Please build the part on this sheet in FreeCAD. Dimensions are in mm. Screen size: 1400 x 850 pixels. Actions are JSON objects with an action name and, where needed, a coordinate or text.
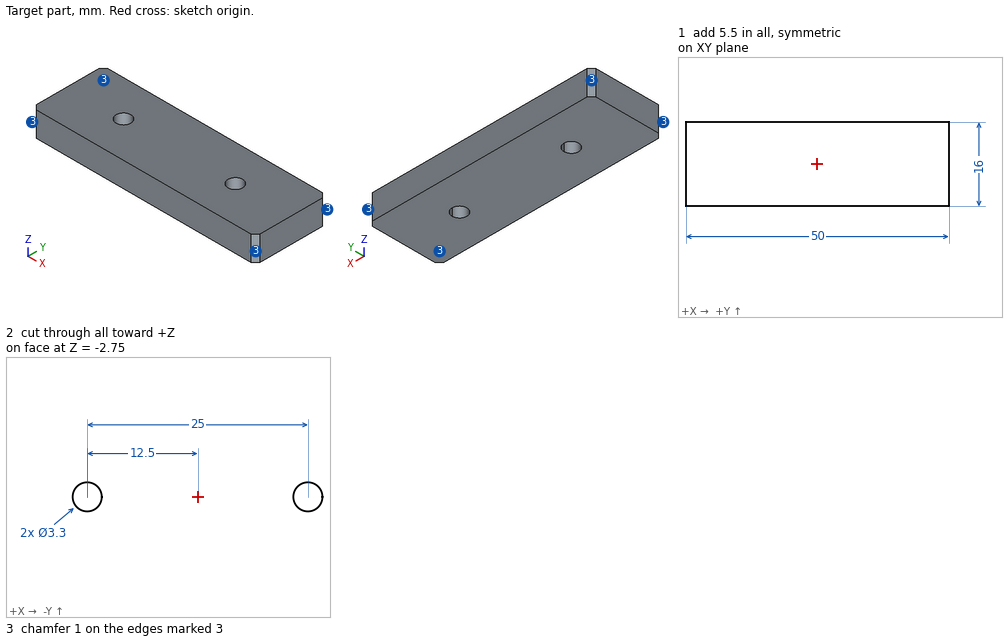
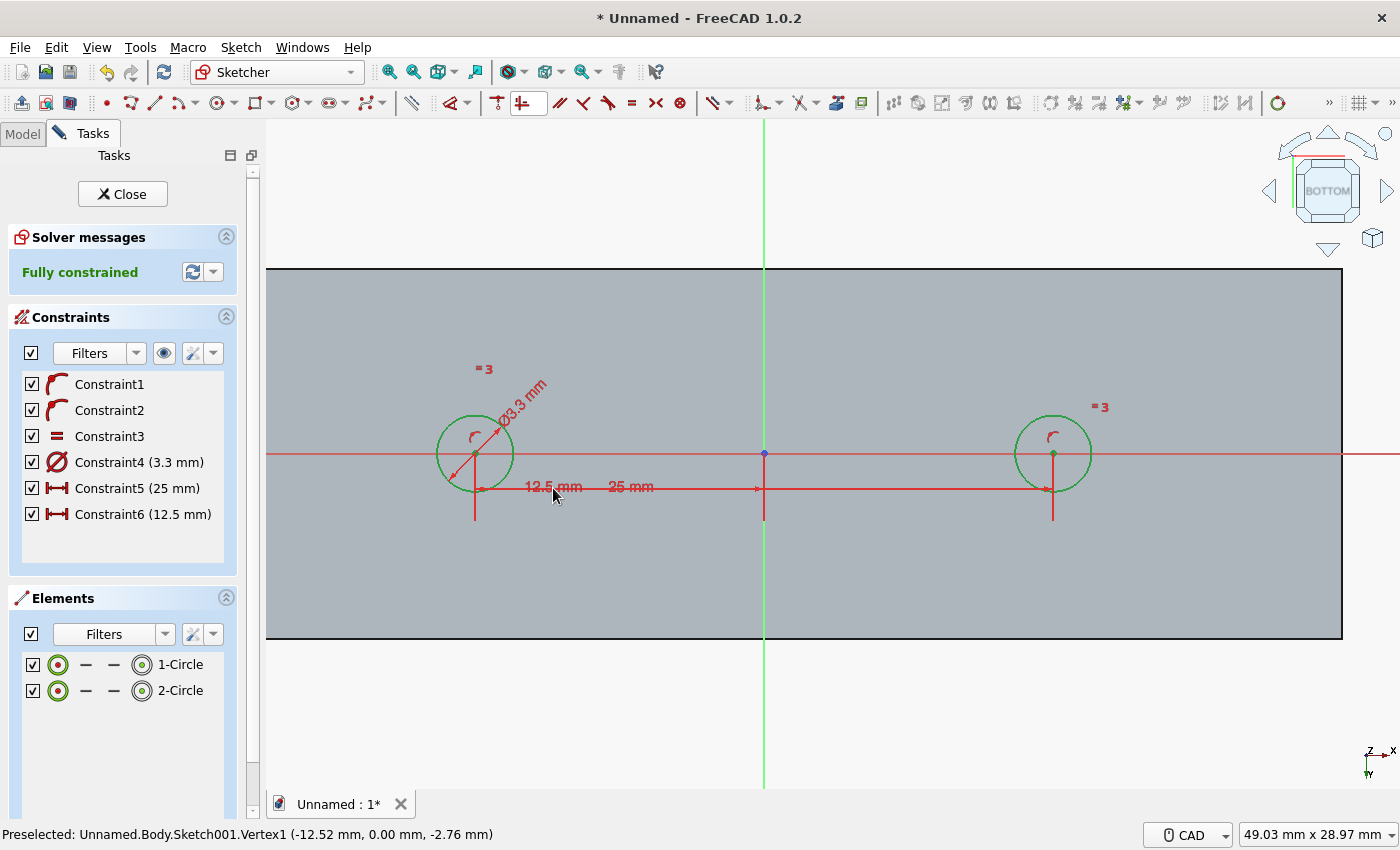
{"action": "left_click", "coordinate": [123, 194]}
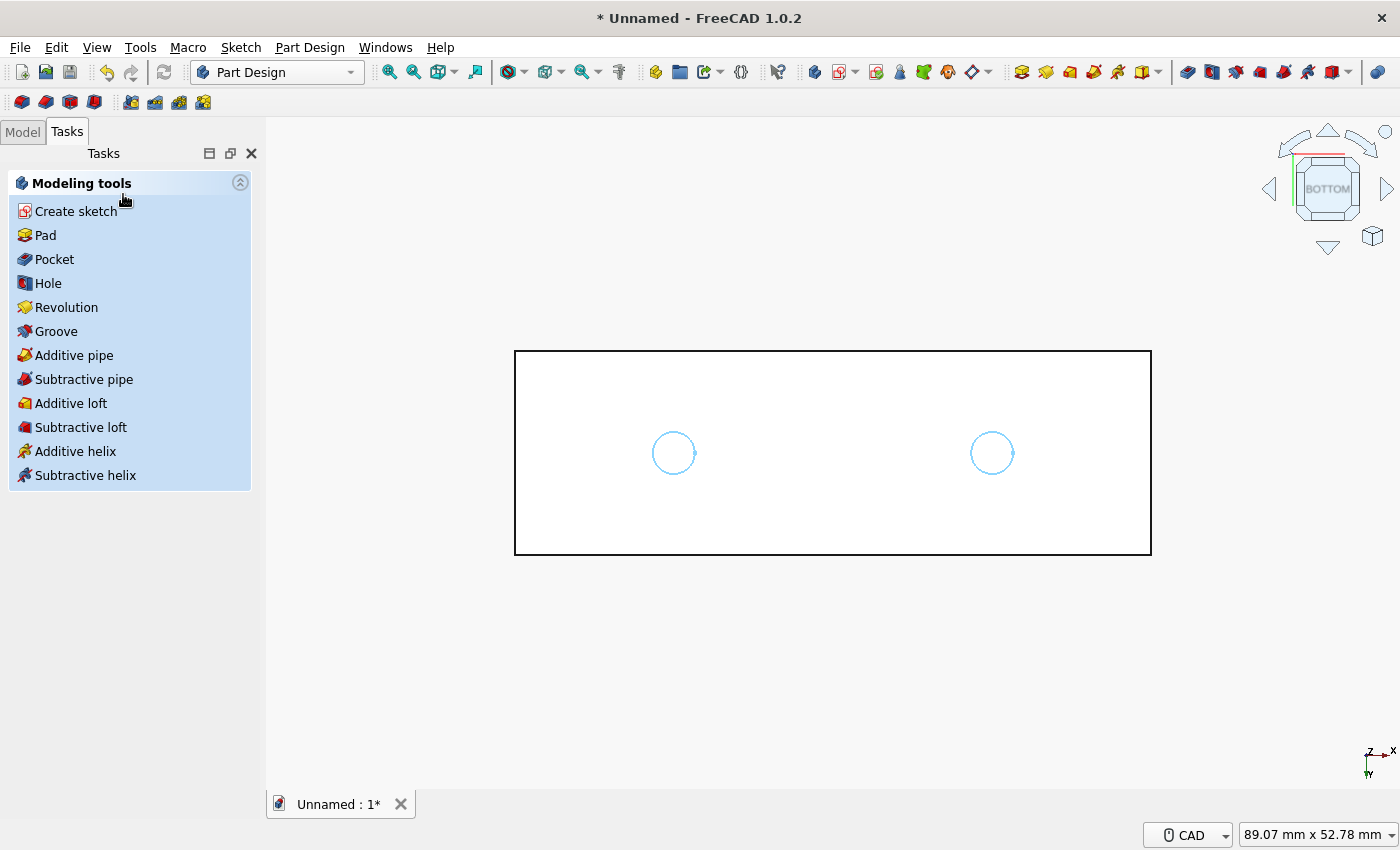
{"action": "left_click", "coordinate": [1188, 72]}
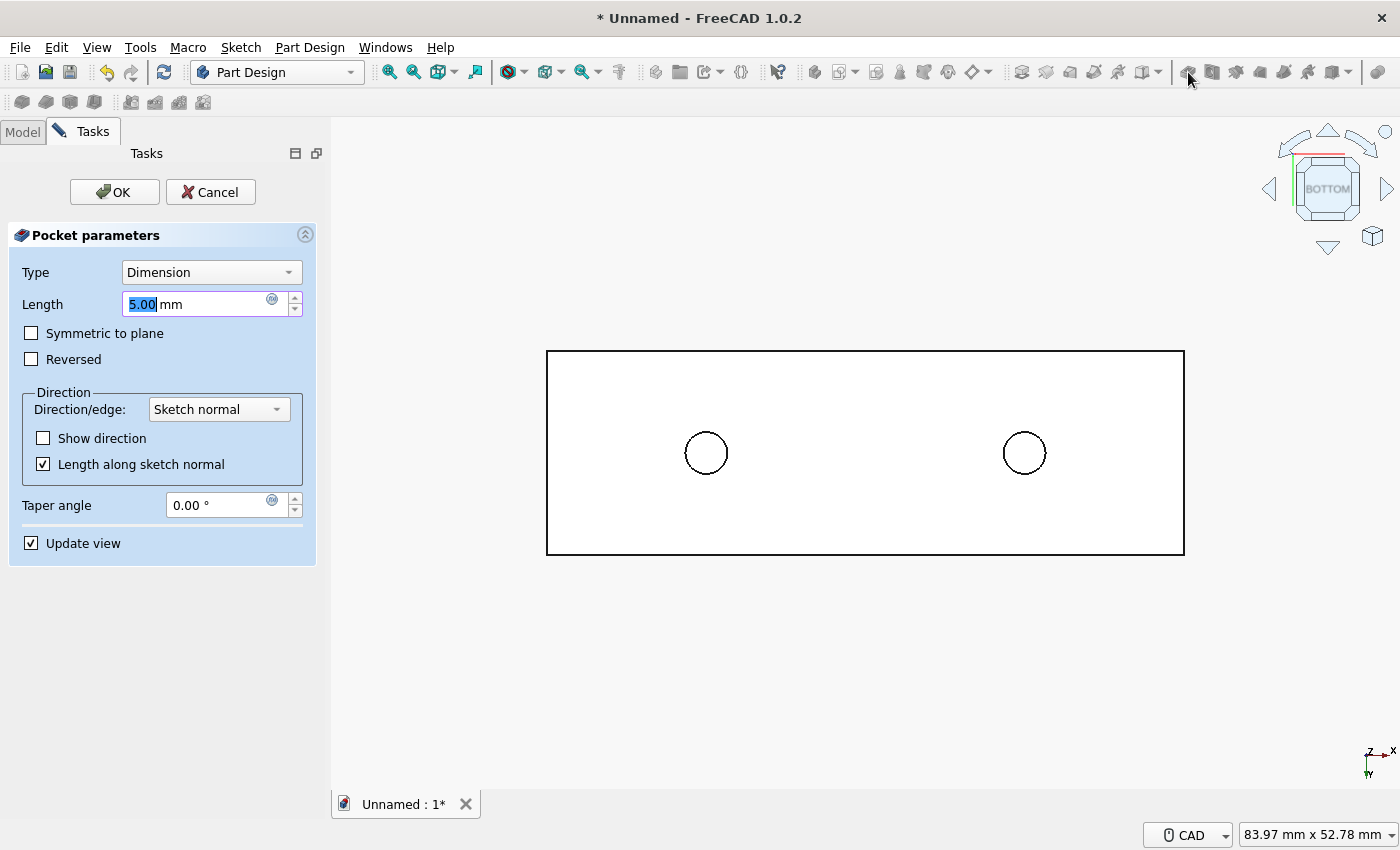
{"action": "left_click", "coordinate": [212, 272]}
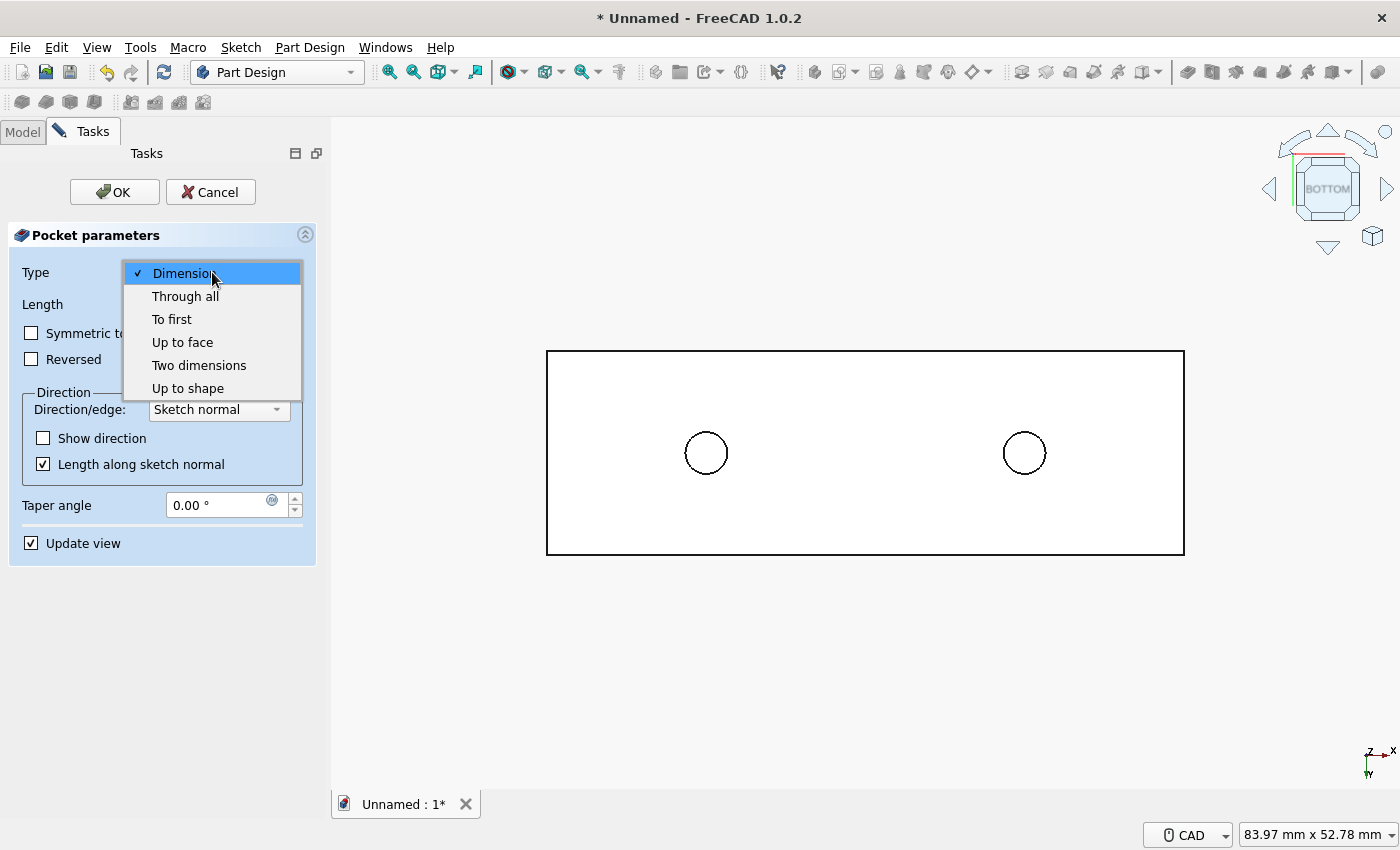
{"action": "left_click", "coordinate": [212, 296]}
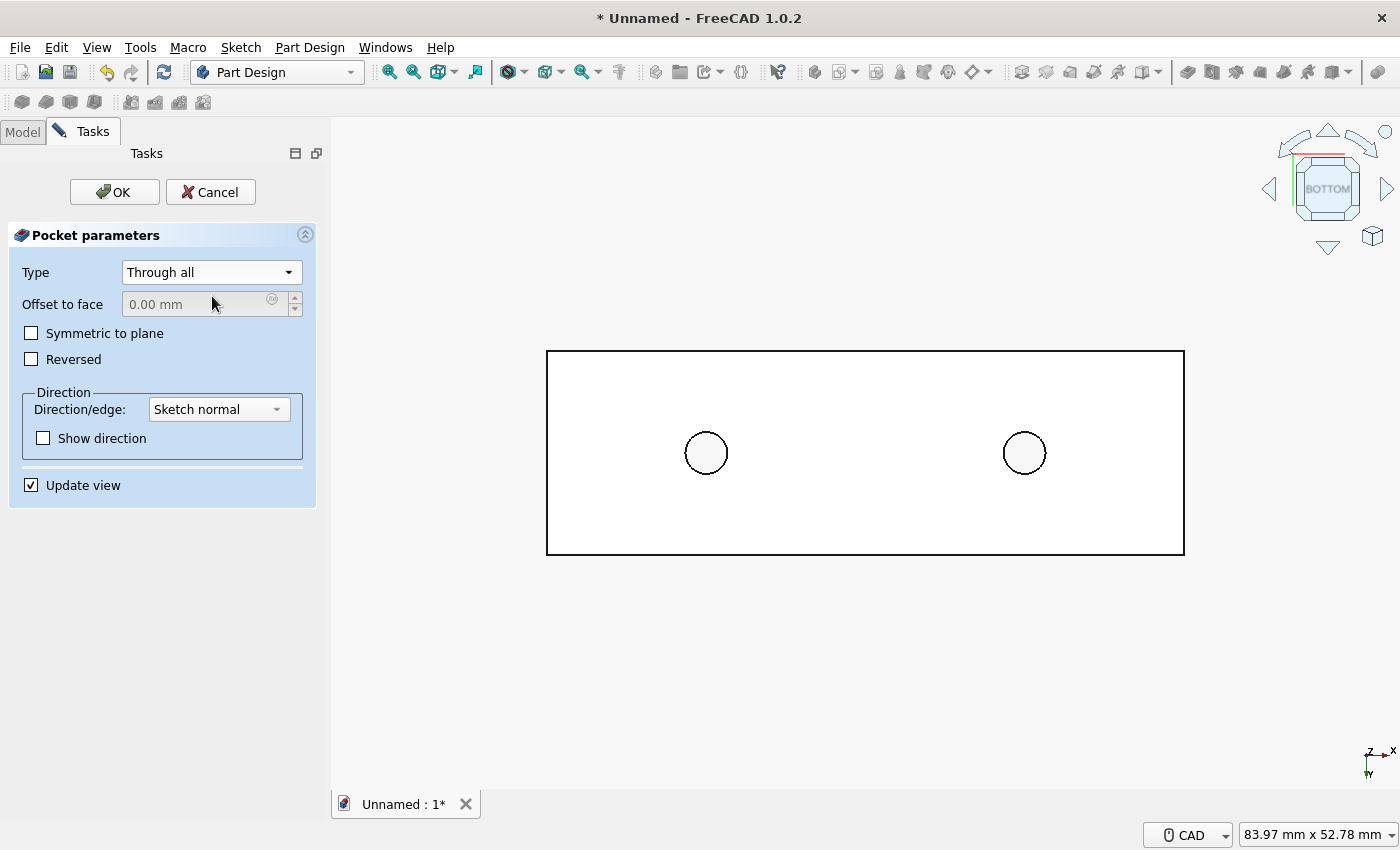
{"action": "left_click", "coordinate": [115, 192]}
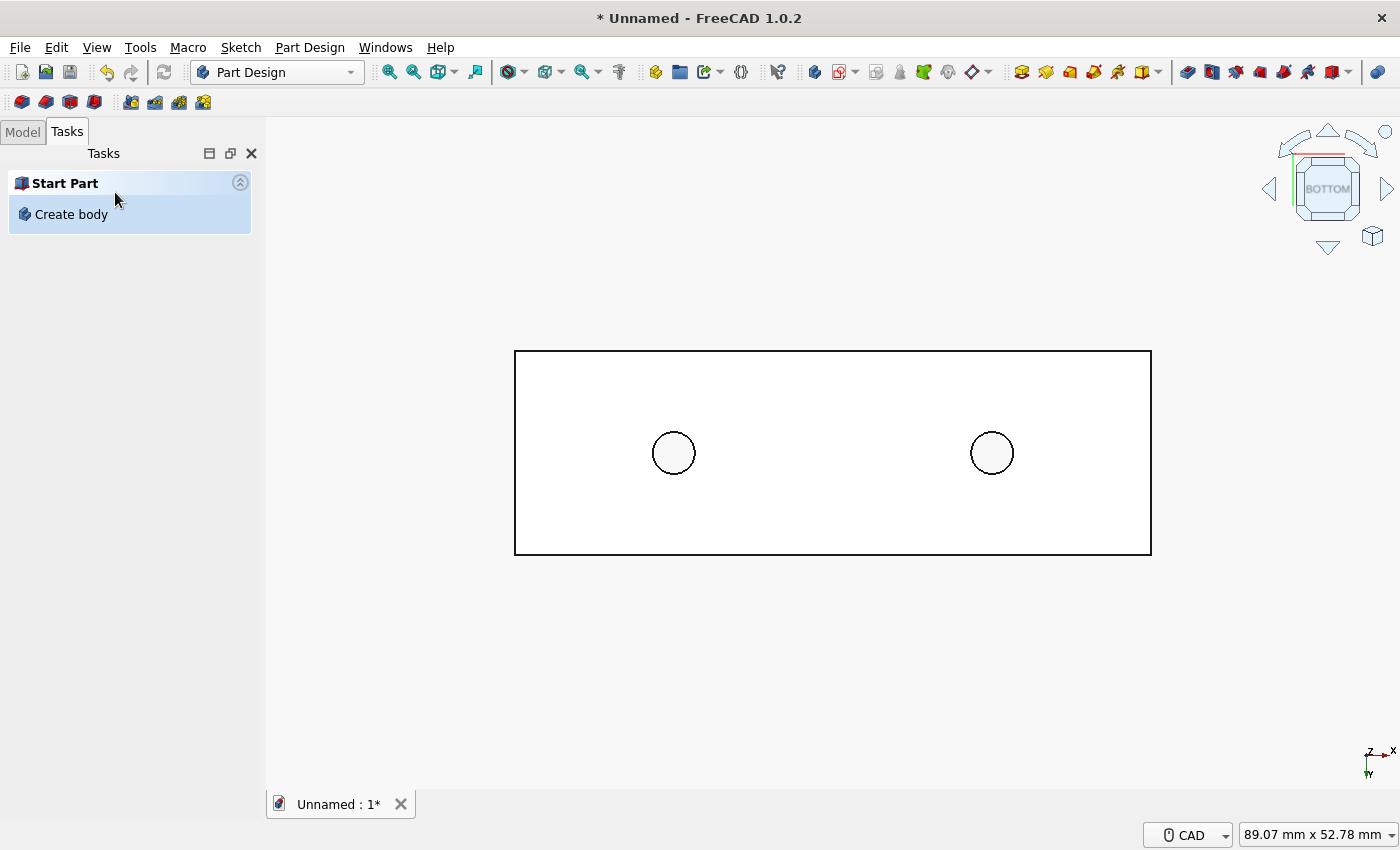
{"action": "key", "text": "0"}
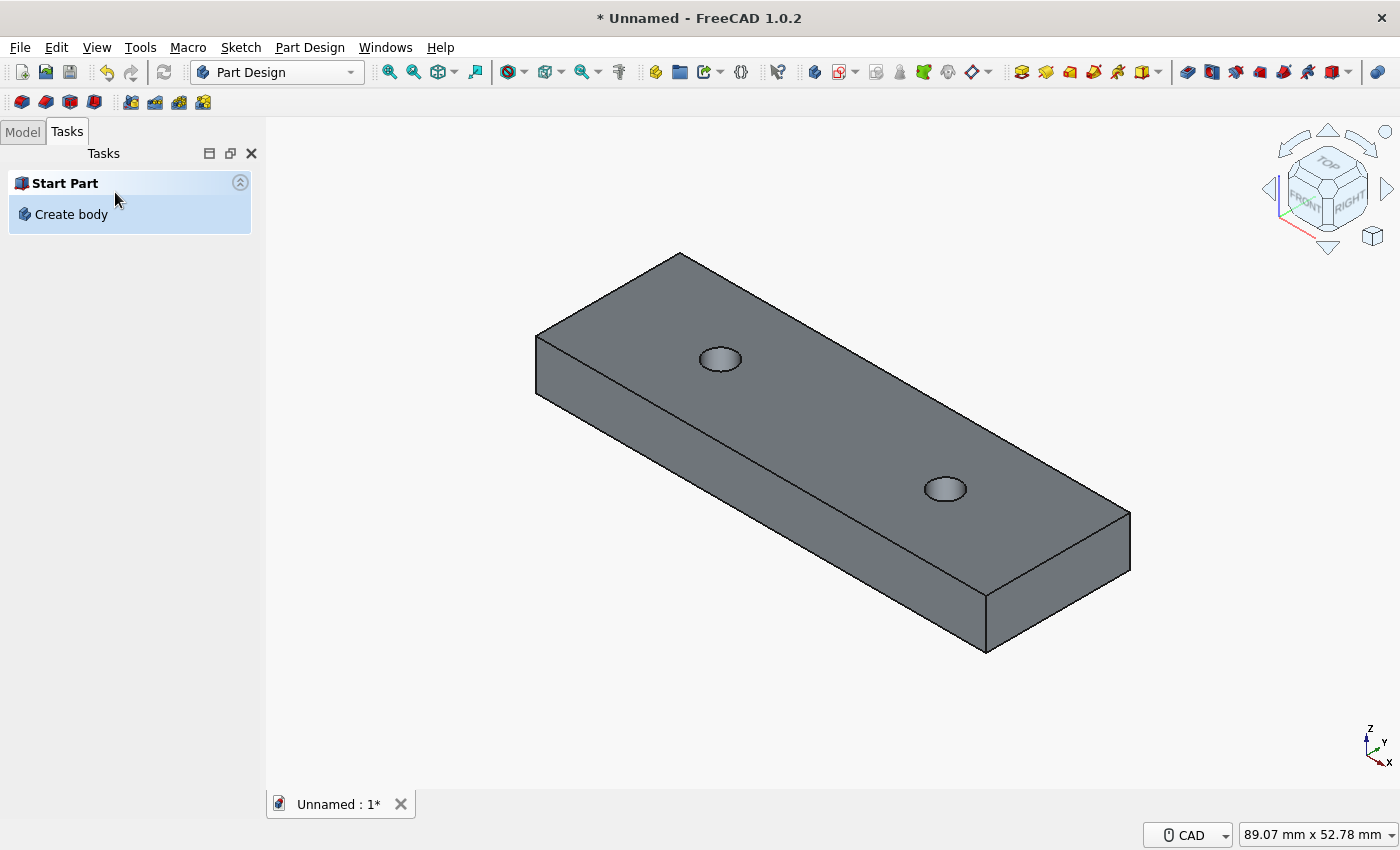
{"action": "left_click", "coordinate": [986, 624]}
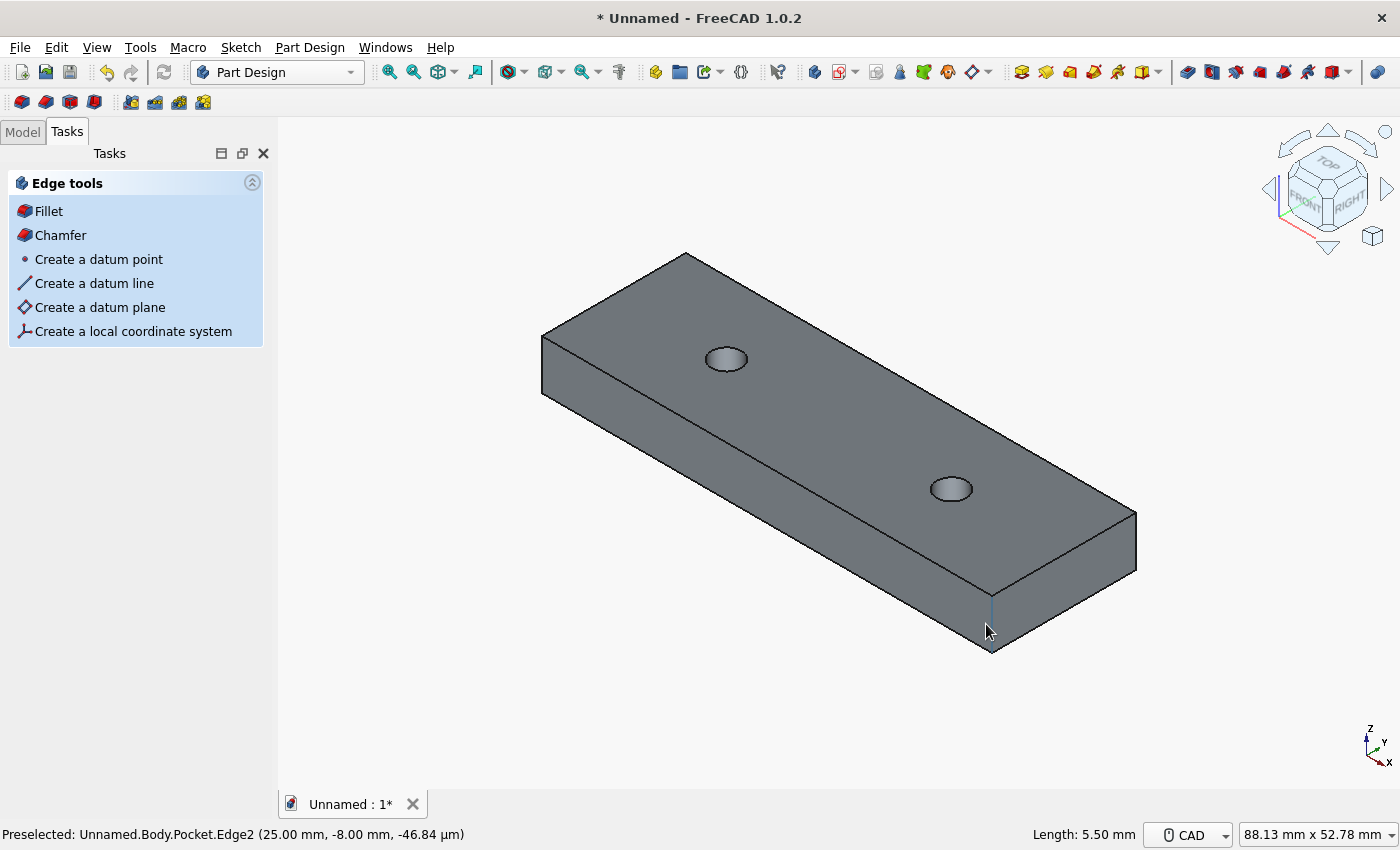
{"action": "key", "text": "2"}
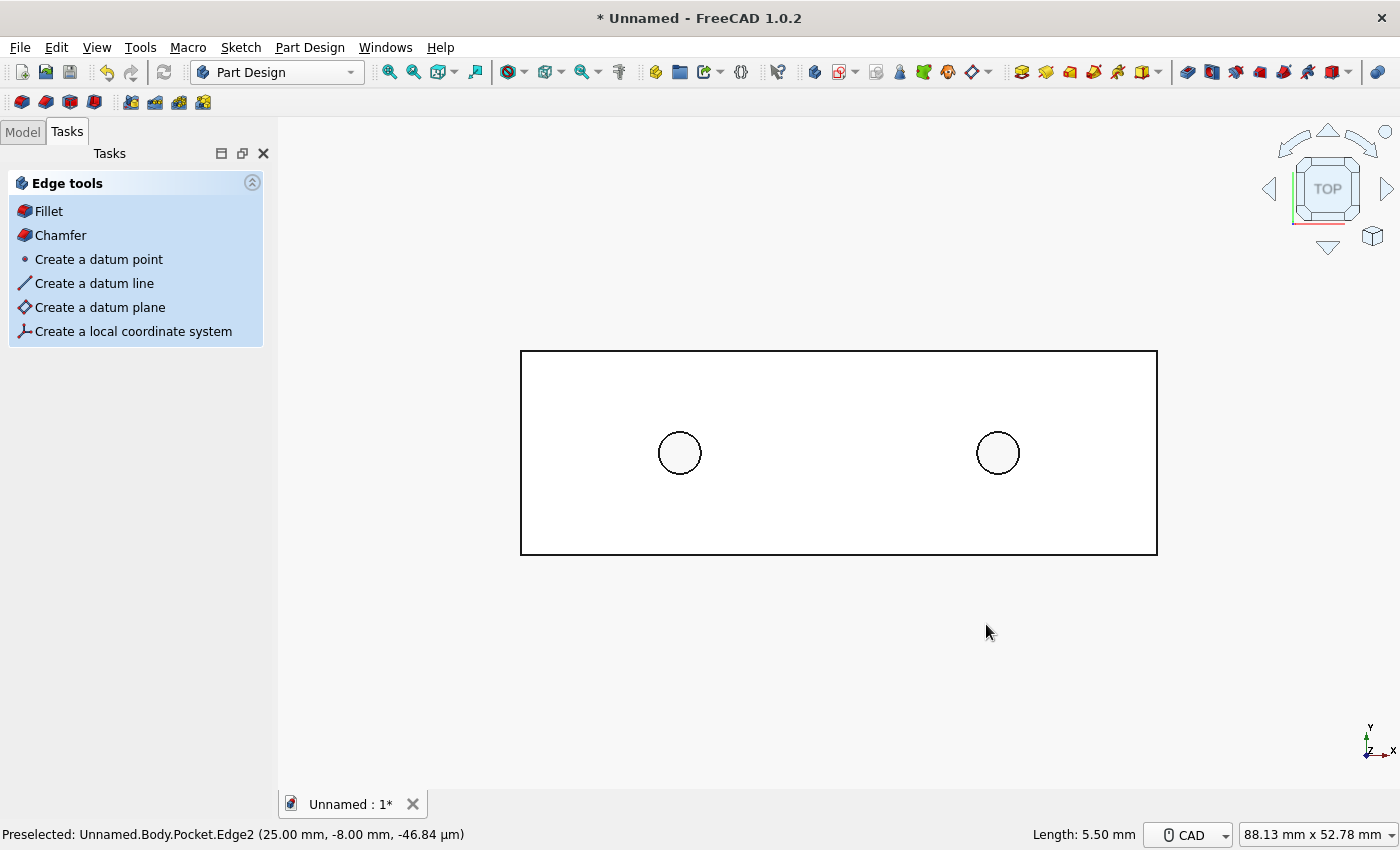
{"action": "key", "text": "1"}